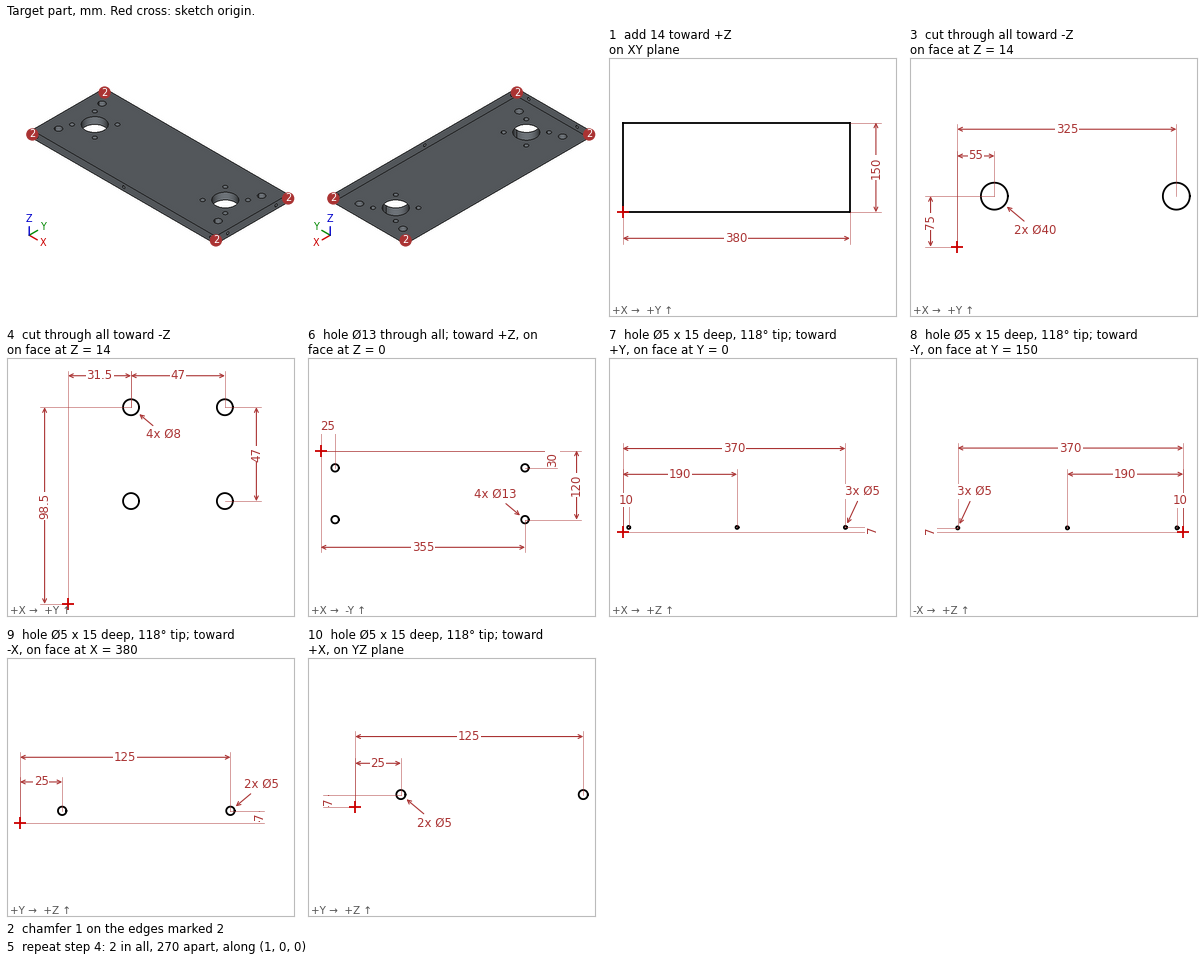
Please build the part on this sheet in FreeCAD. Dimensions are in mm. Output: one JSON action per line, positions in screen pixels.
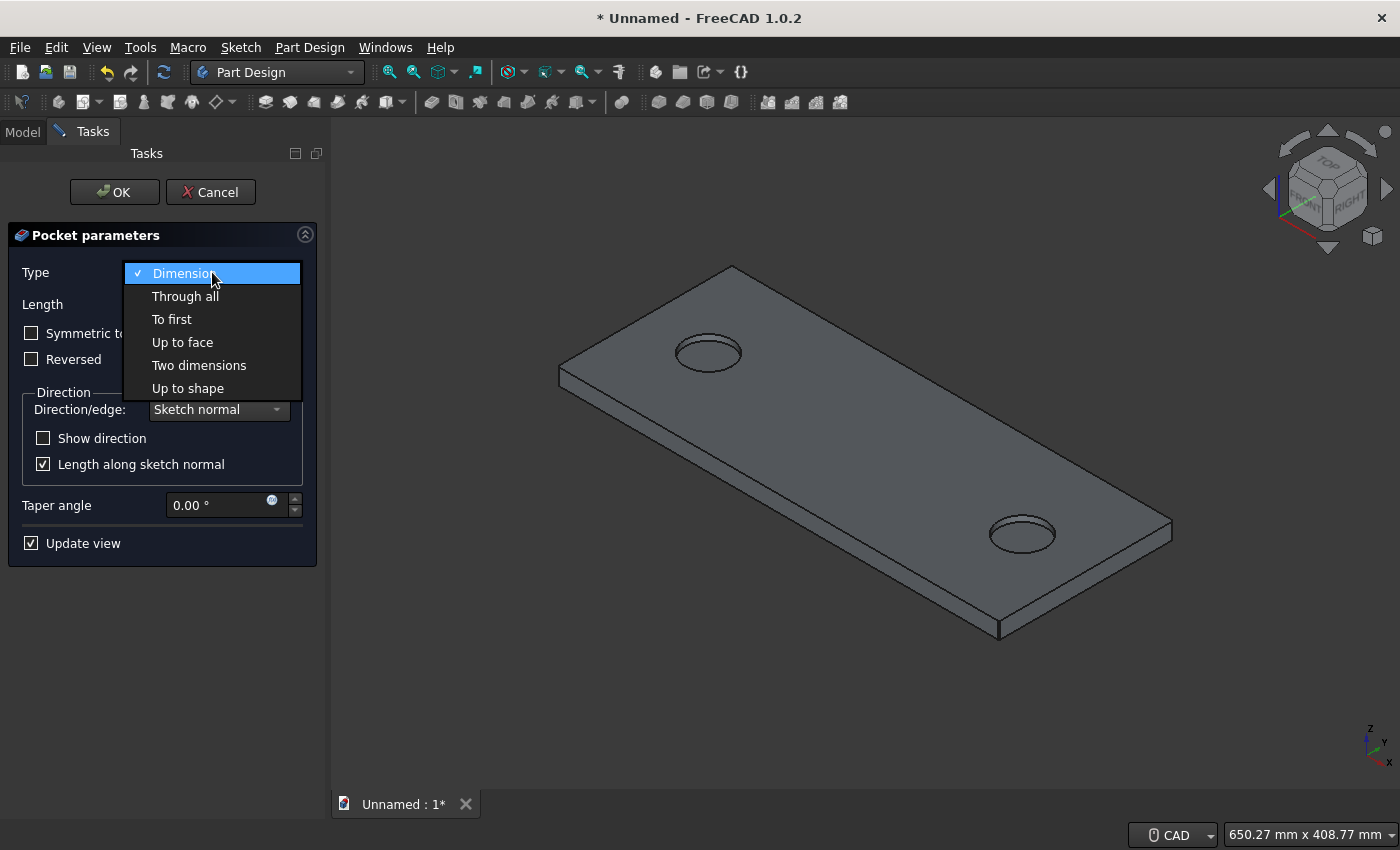
{"action": "left_click", "coordinate": [212, 296]}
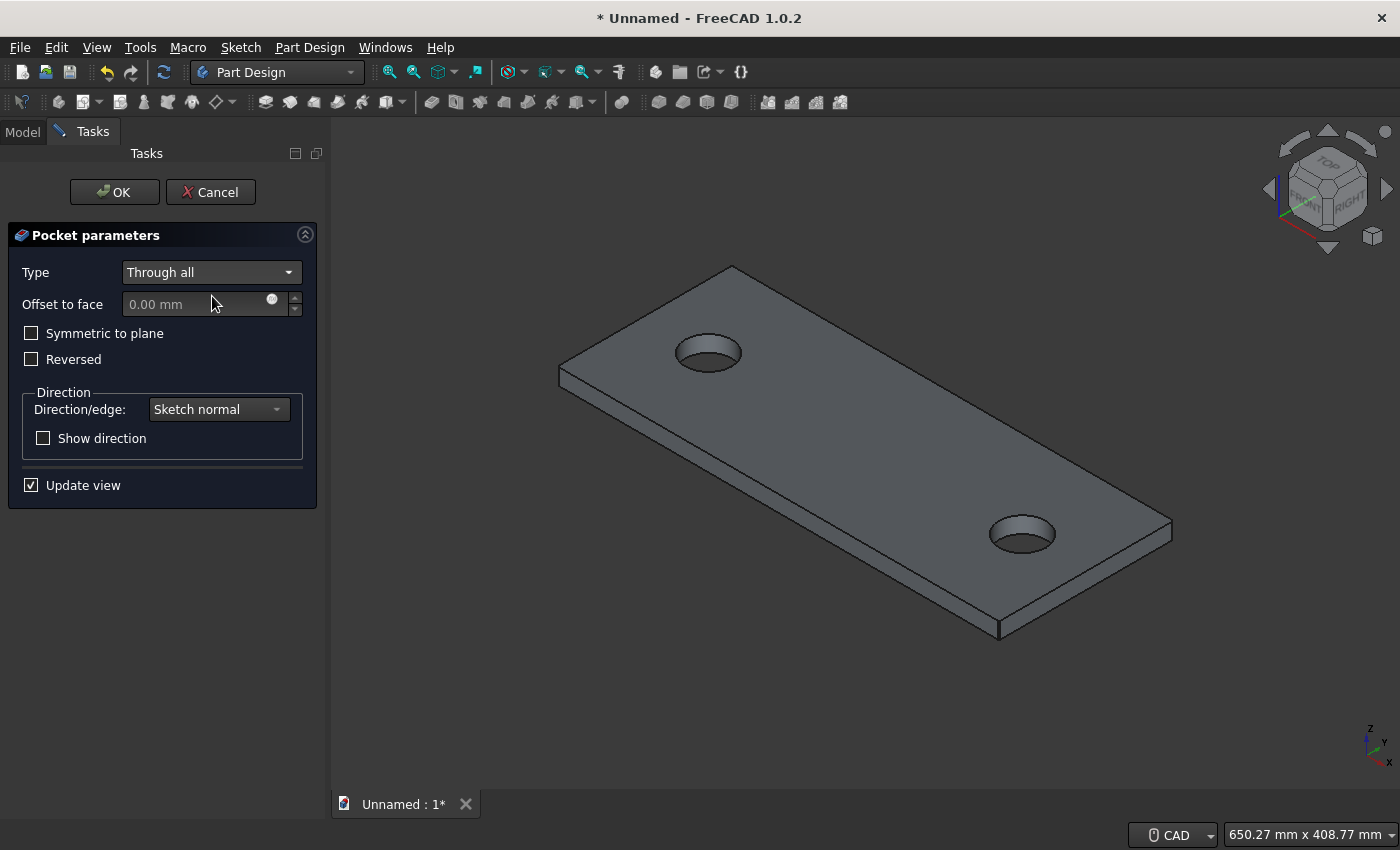
{"action": "left_click", "coordinate": [115, 192]}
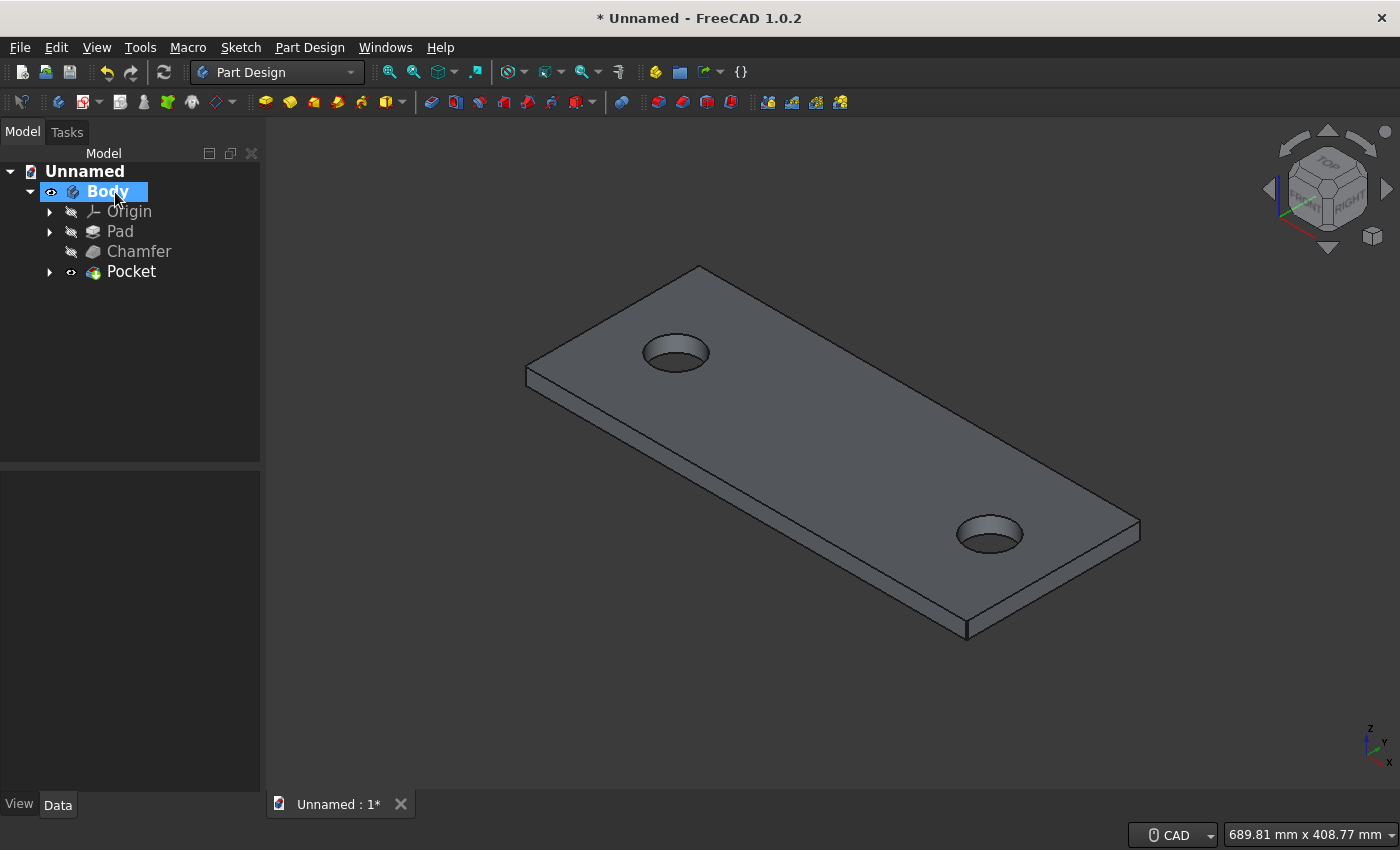
{"action": "left_click", "coordinate": [833, 443]}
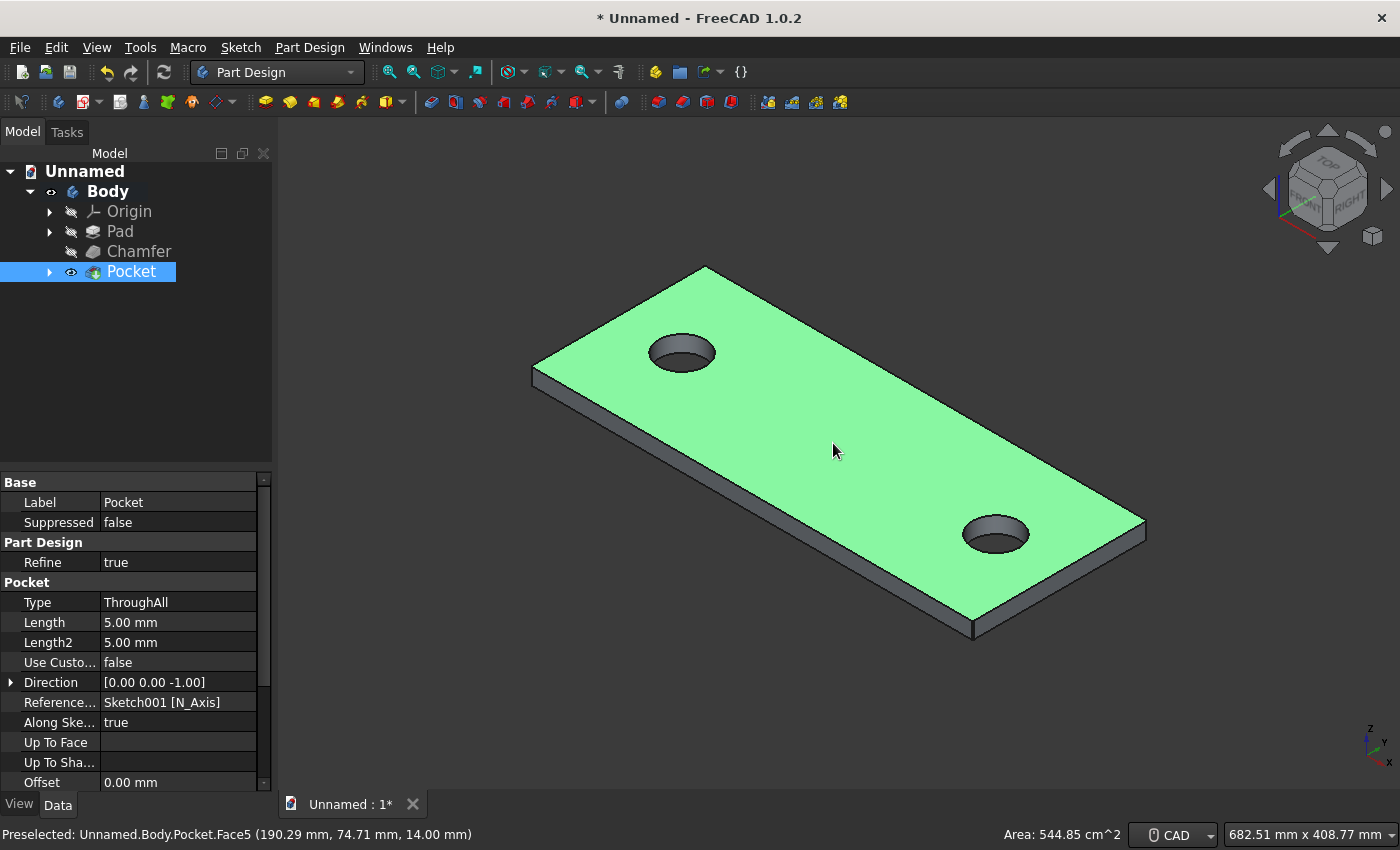
{"action": "left_click", "coordinate": [84, 102]}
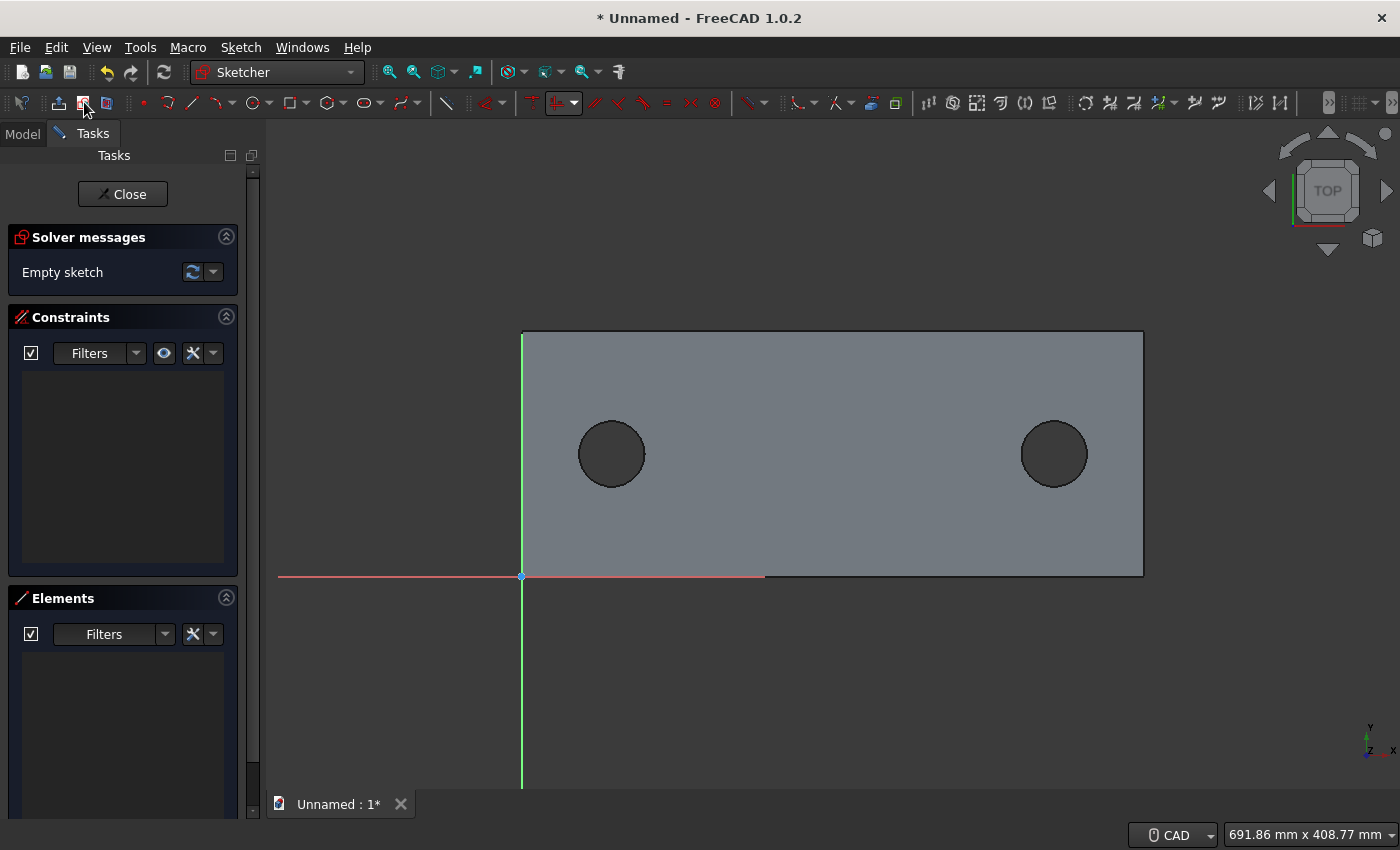
{"action": "scroll", "coordinate": [487, 516], "scroll_direction": "up", "scroll_amount": 5}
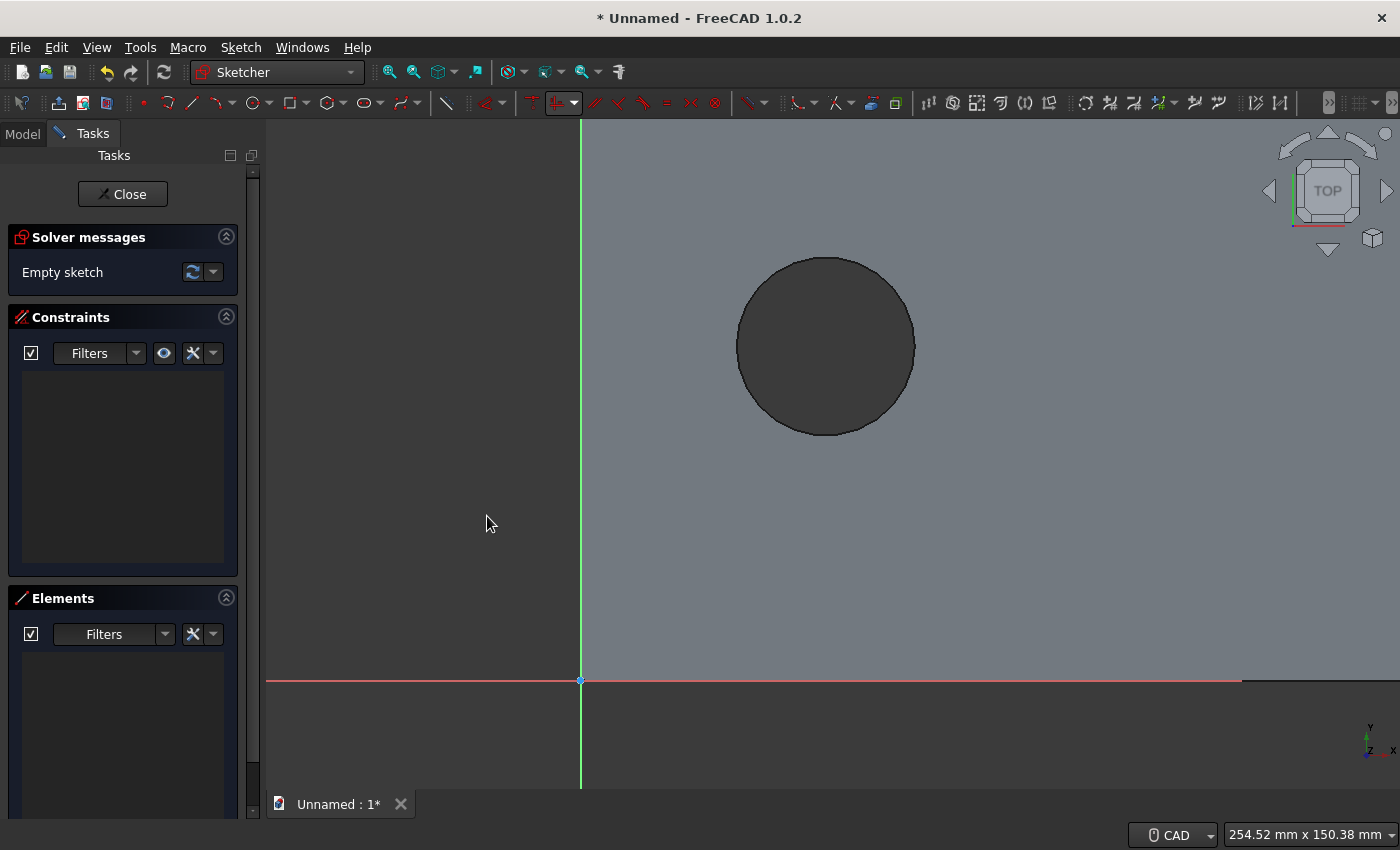
{"action": "key", "text": "g c"}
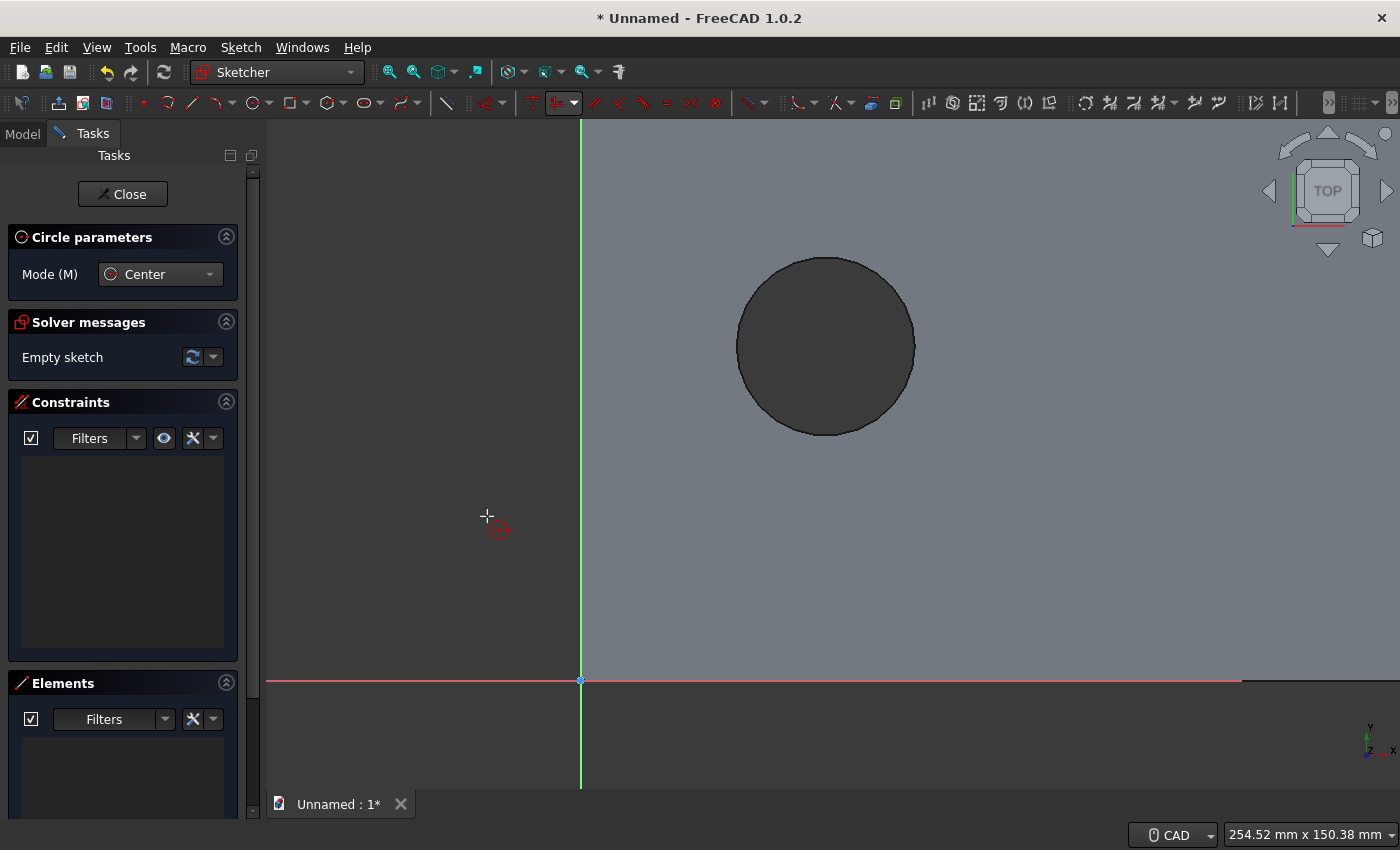
{"action": "scroll", "coordinate": [721, 242], "scroll_direction": "up", "scroll_amount": 2}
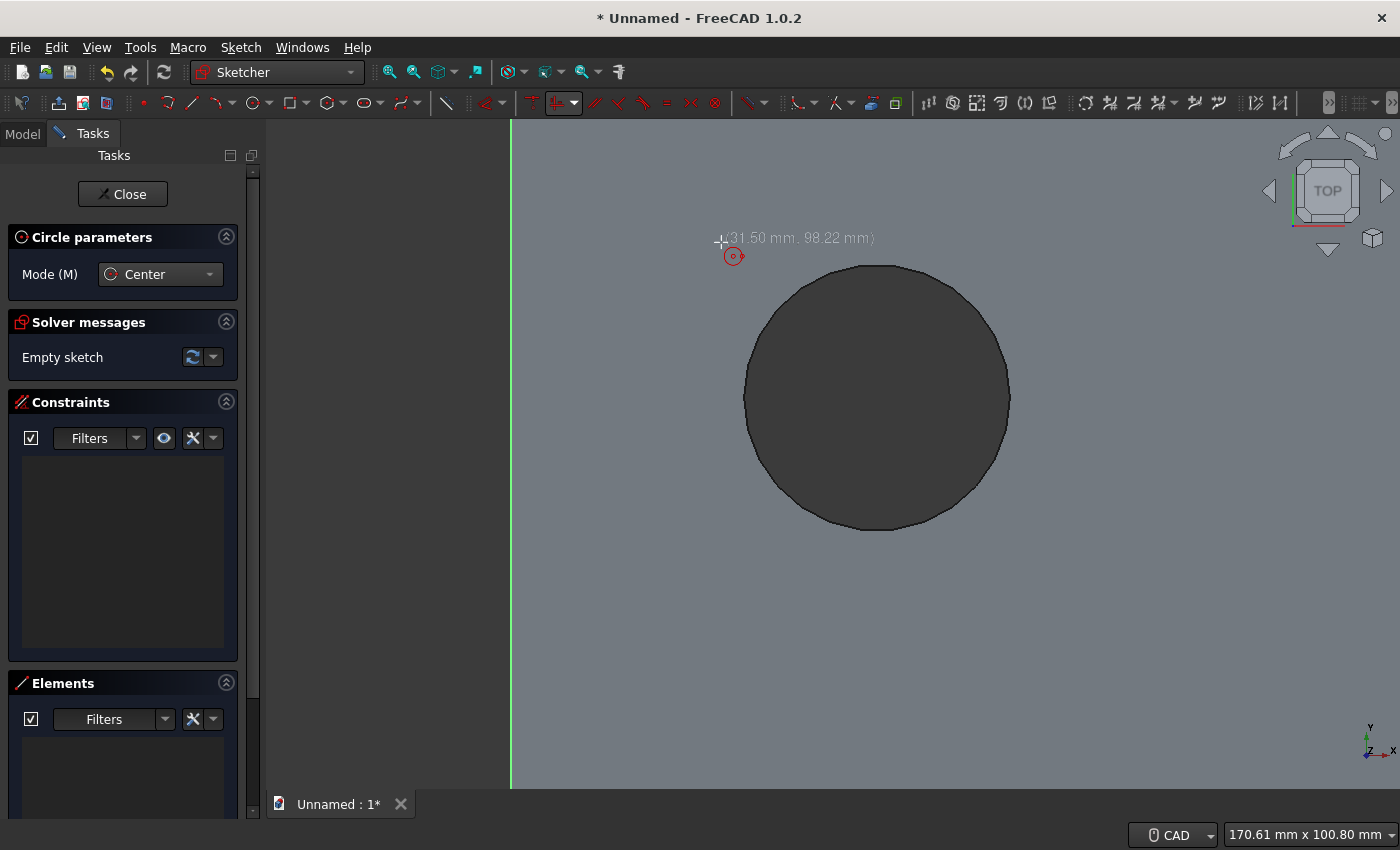
{"action": "left_click", "coordinate": [721, 242]}
{"action": "mouse_move", "coordinate": [740, 223]}